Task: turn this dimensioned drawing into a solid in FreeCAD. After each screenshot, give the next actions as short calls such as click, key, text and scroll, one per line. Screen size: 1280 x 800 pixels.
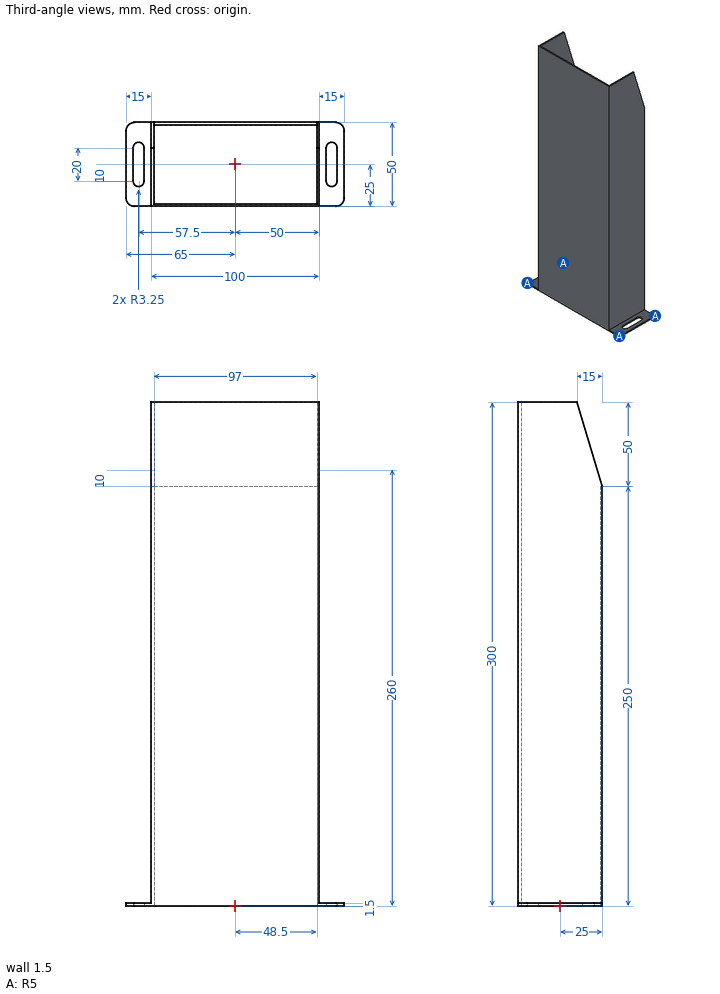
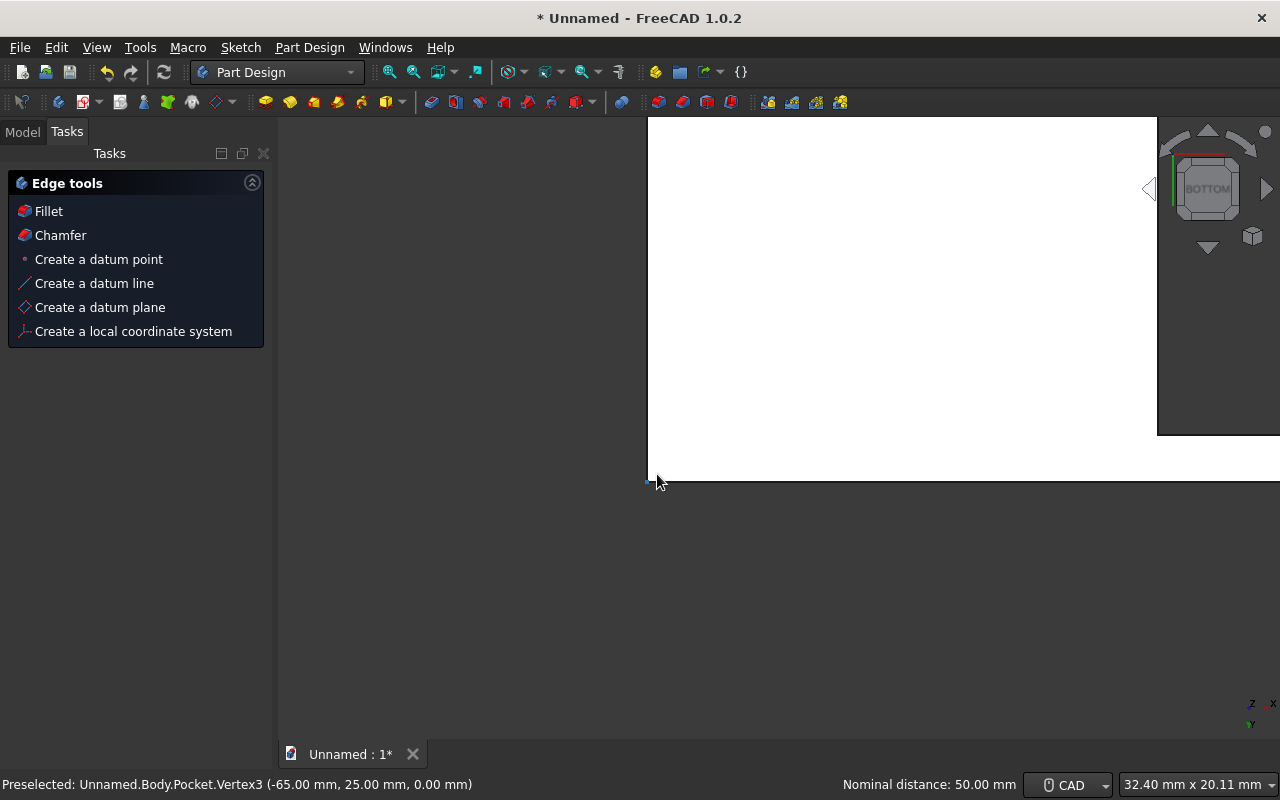
click(390, 72)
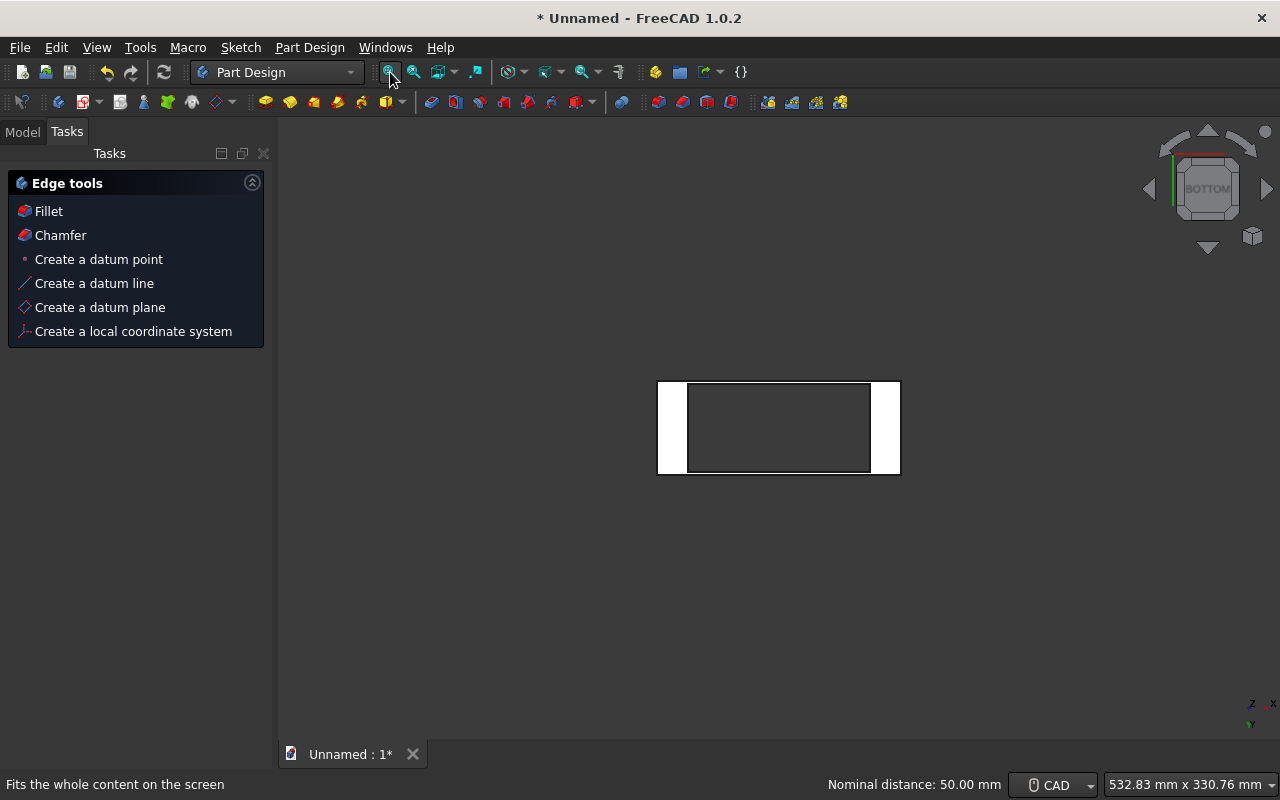
key(4)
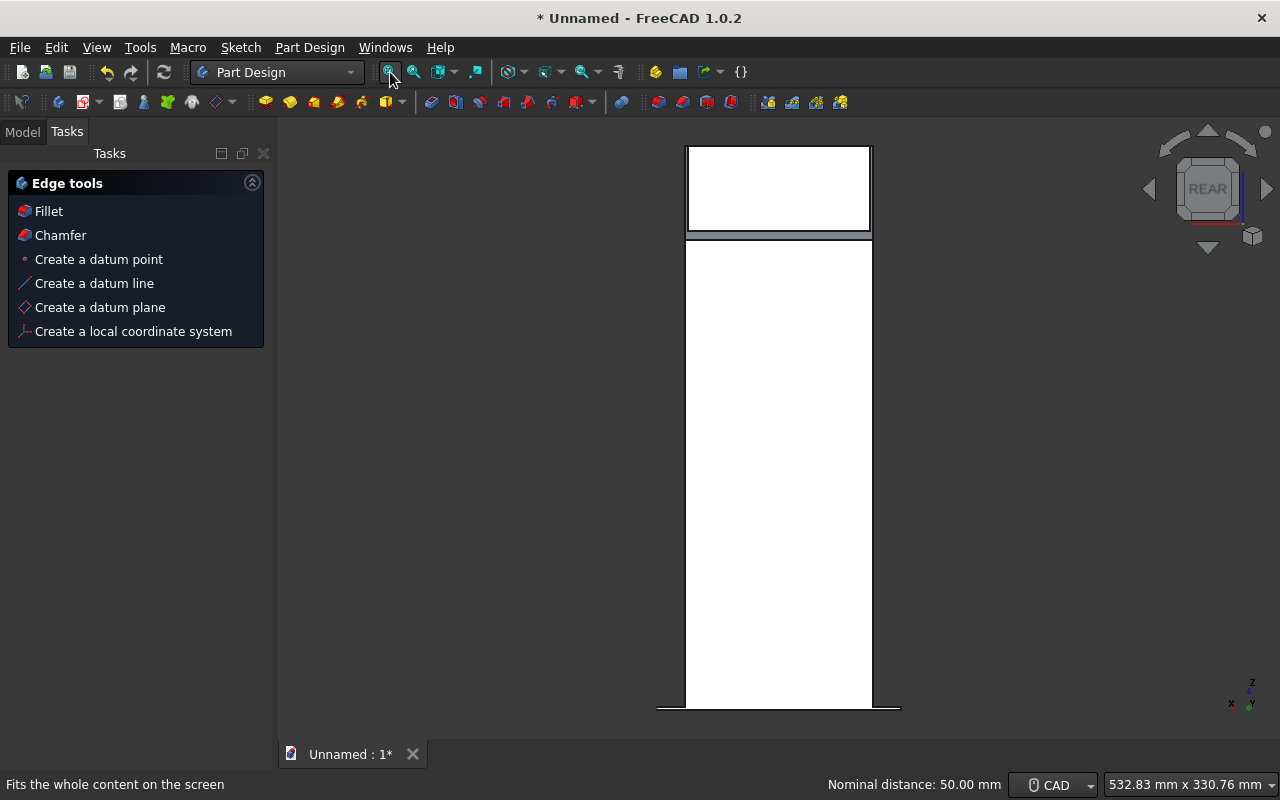
scroll(901, 708, up, 14)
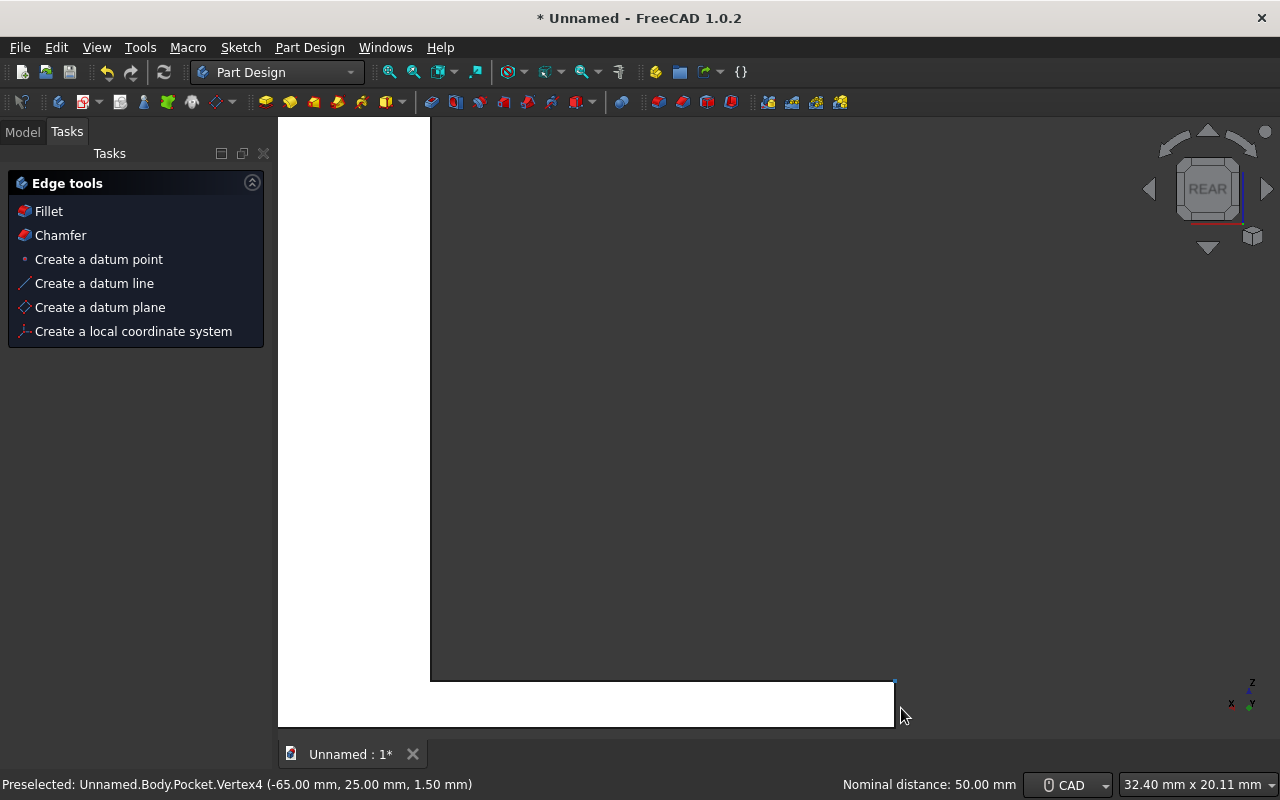
click(895, 703, ctrl)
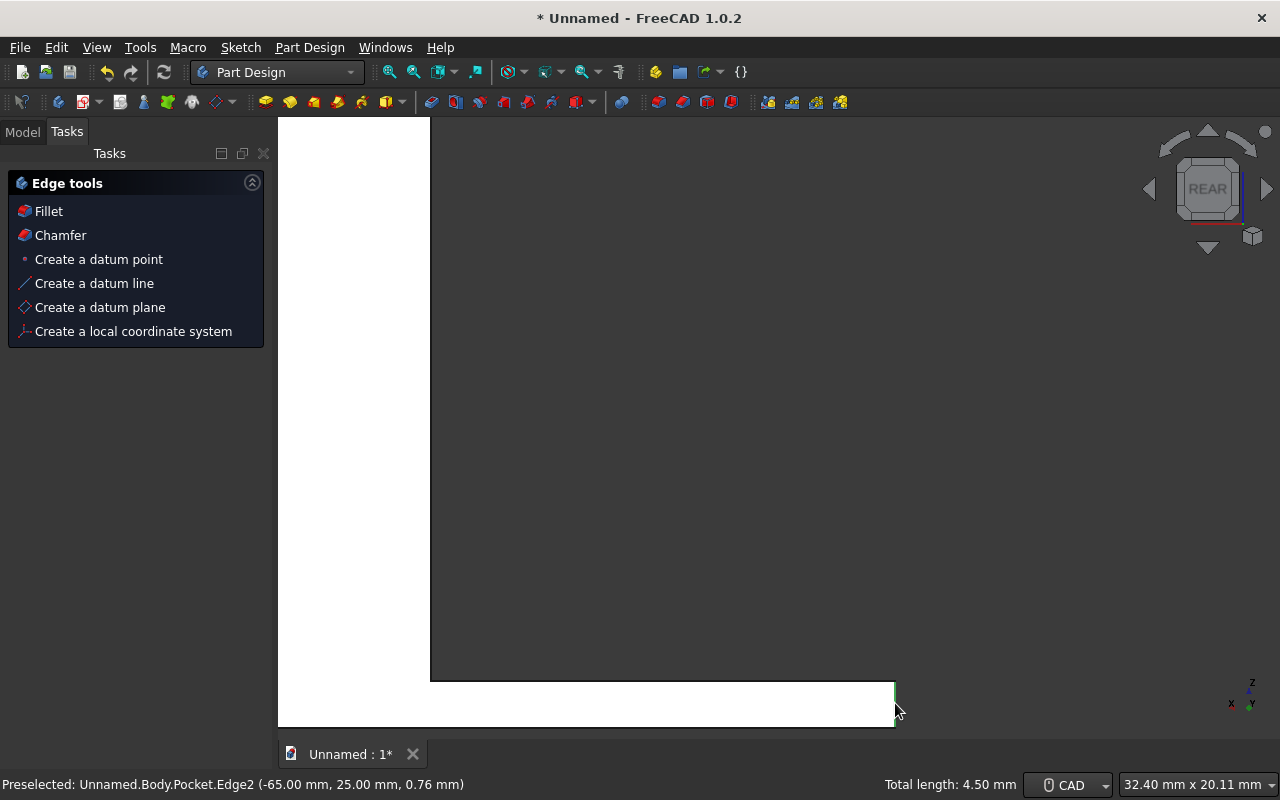
click(390, 72)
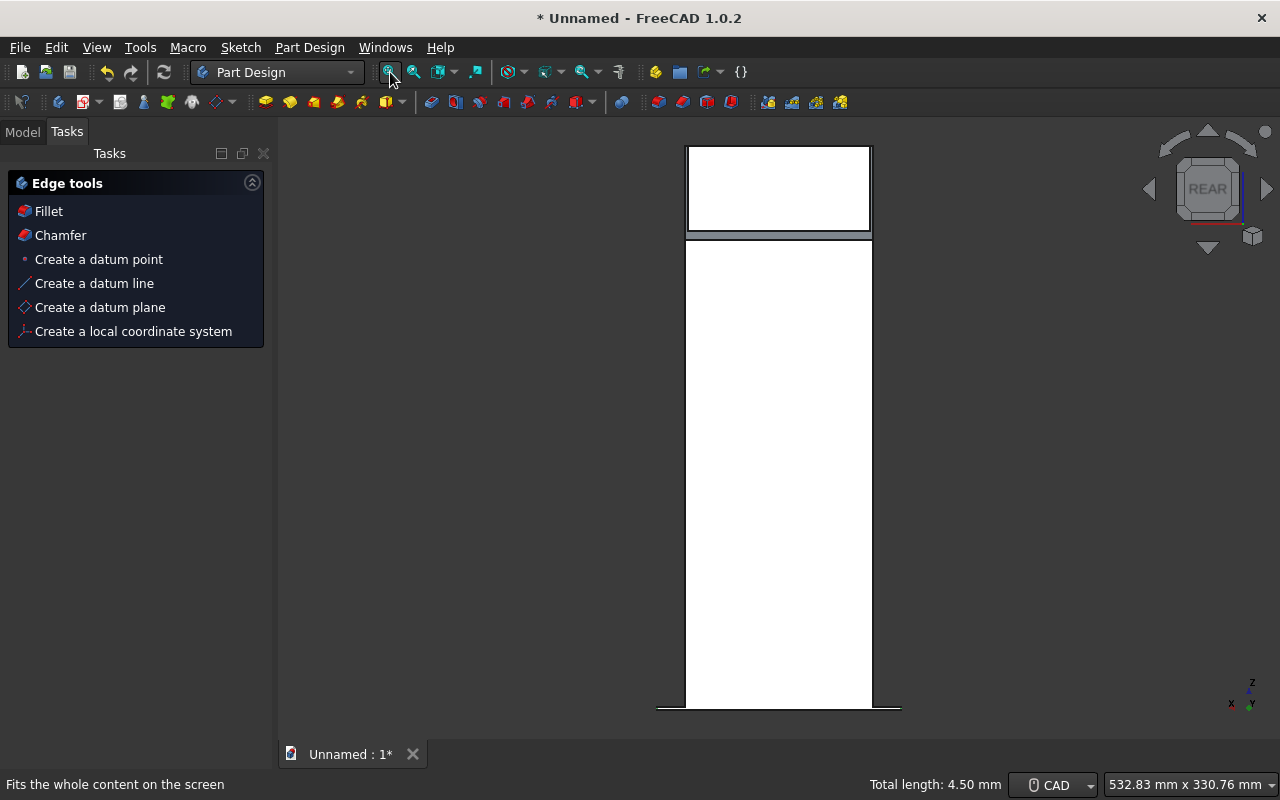
key(6)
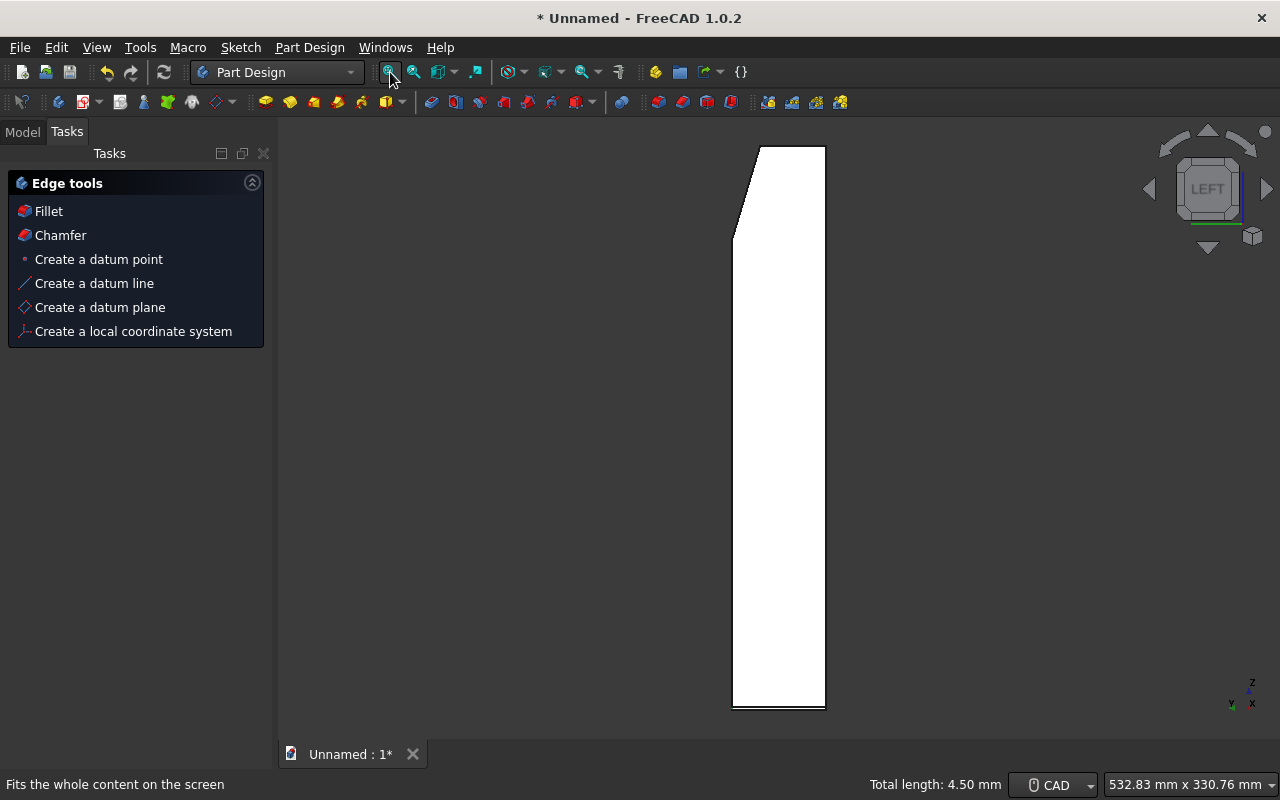
scroll(826, 708, up, 14)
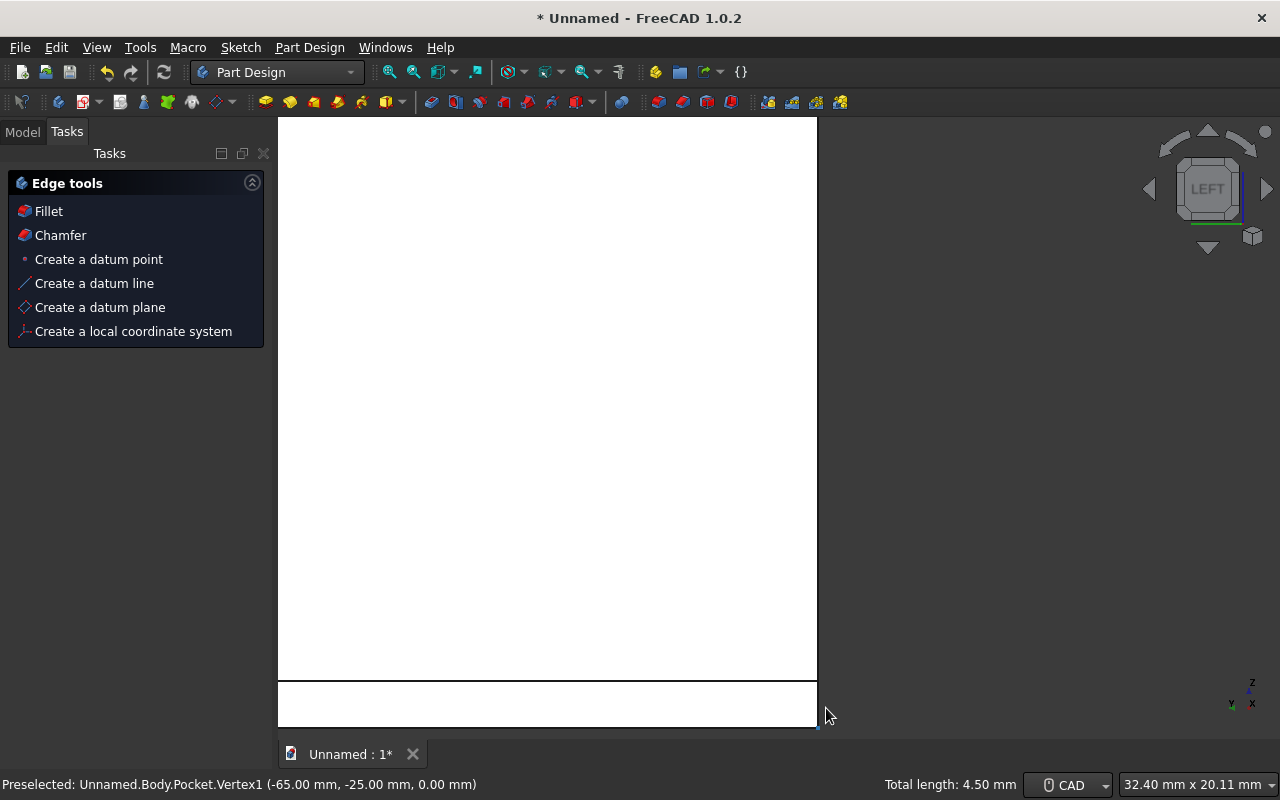
click(818, 703, ctrl)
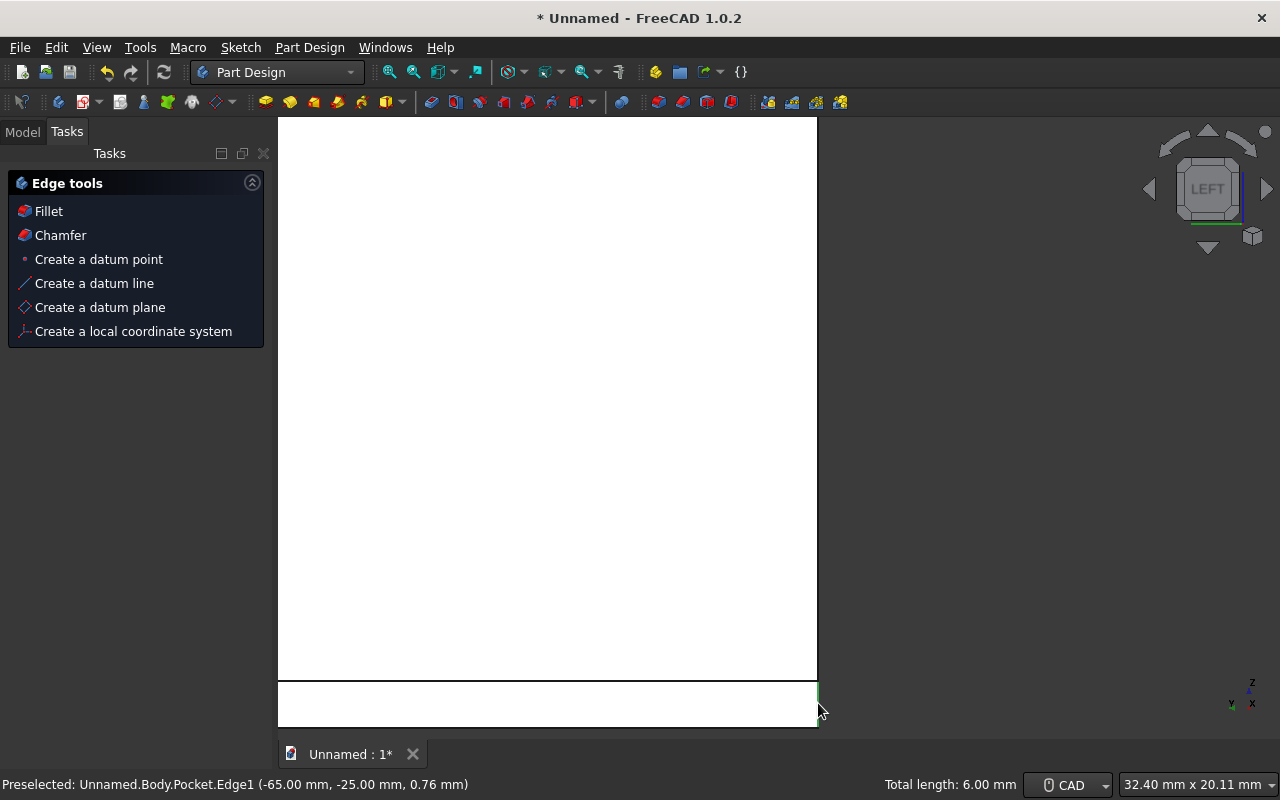
click(660, 102)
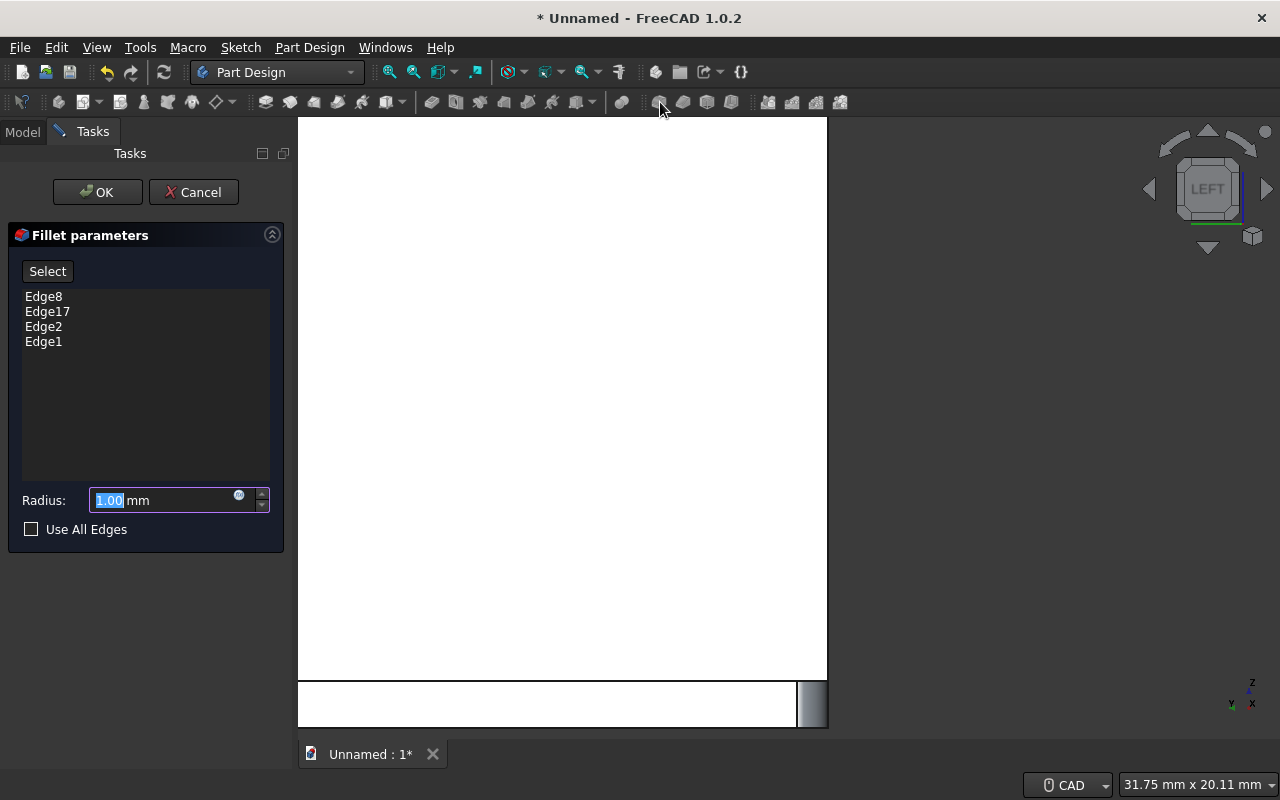
text(5)
key(Tab)